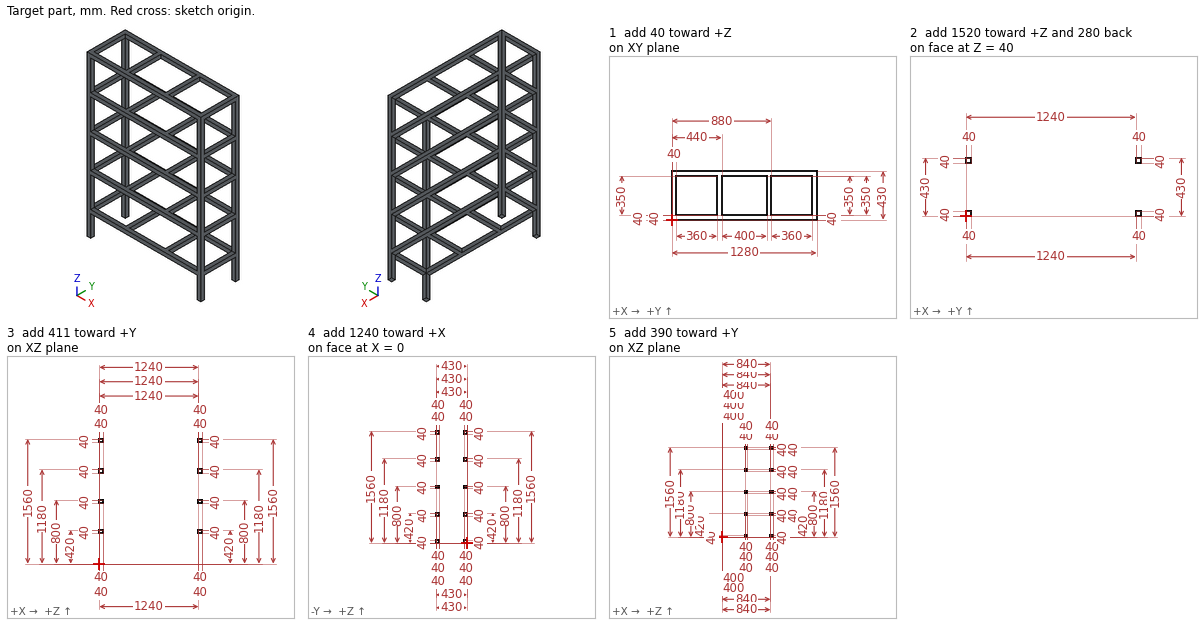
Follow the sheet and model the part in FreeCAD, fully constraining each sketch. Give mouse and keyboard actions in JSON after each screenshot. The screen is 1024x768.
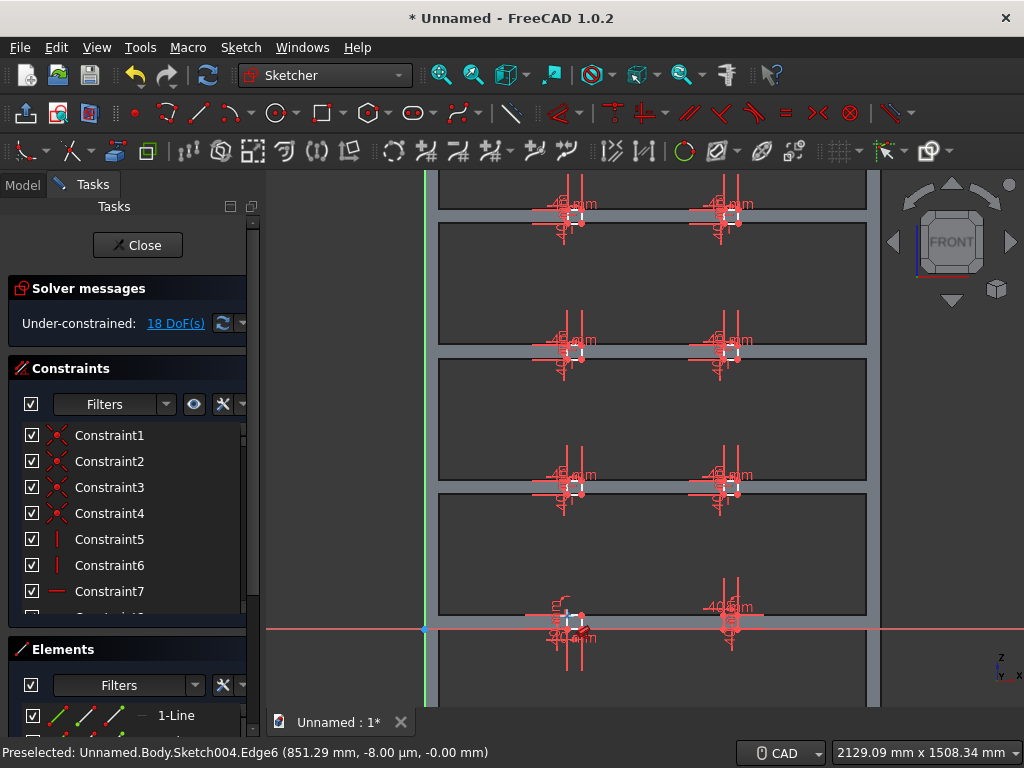
{"action": "left_click", "coordinate": [567, 615]}
{"action": "left_click", "coordinate": [496, 663]}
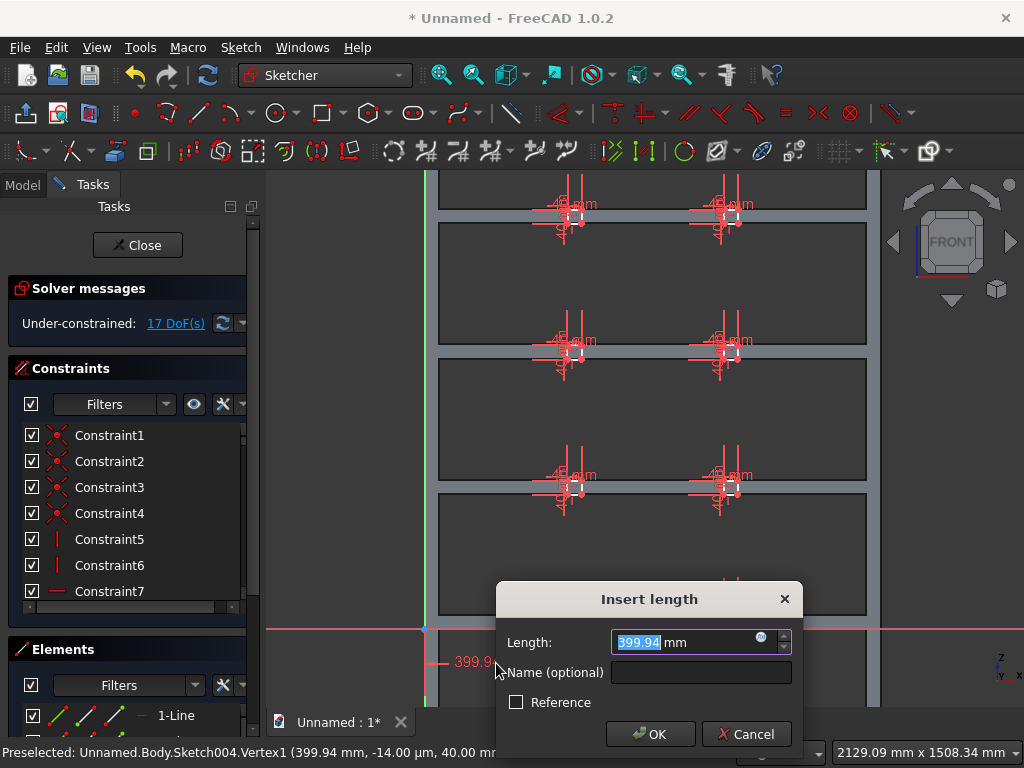
{"action": "type", "text": "400"}
{"action": "key", "text": "Return"}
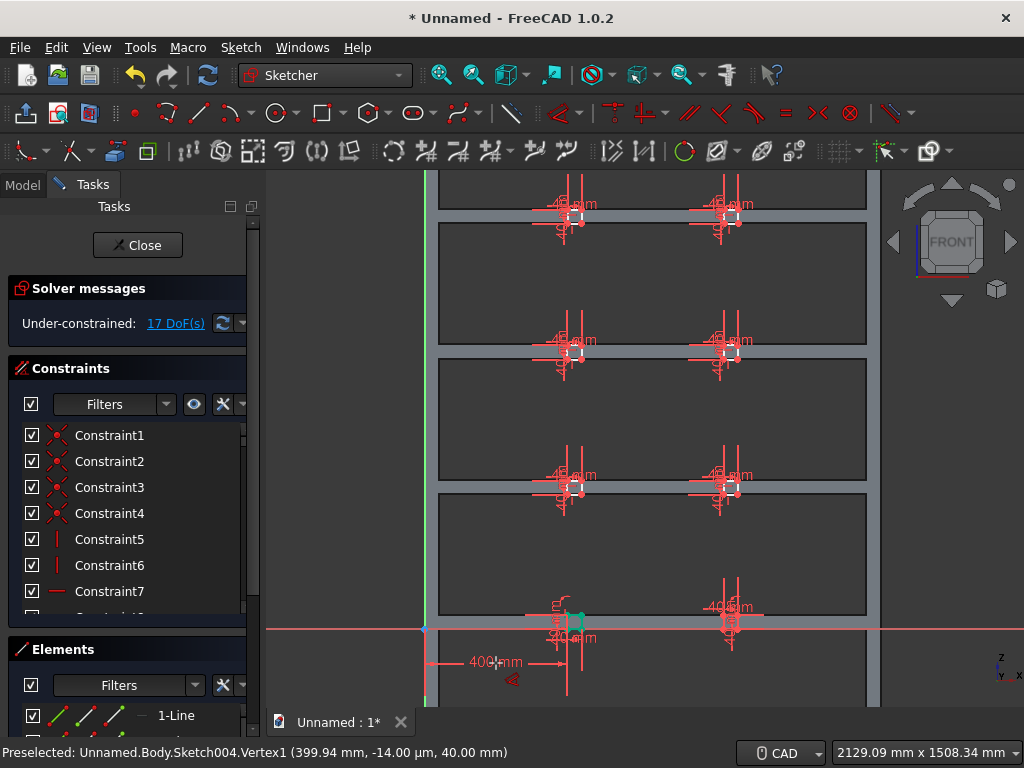
{"action": "left_click", "coordinate": [724, 615]}
{"action": "left_click", "coordinate": [574, 663]}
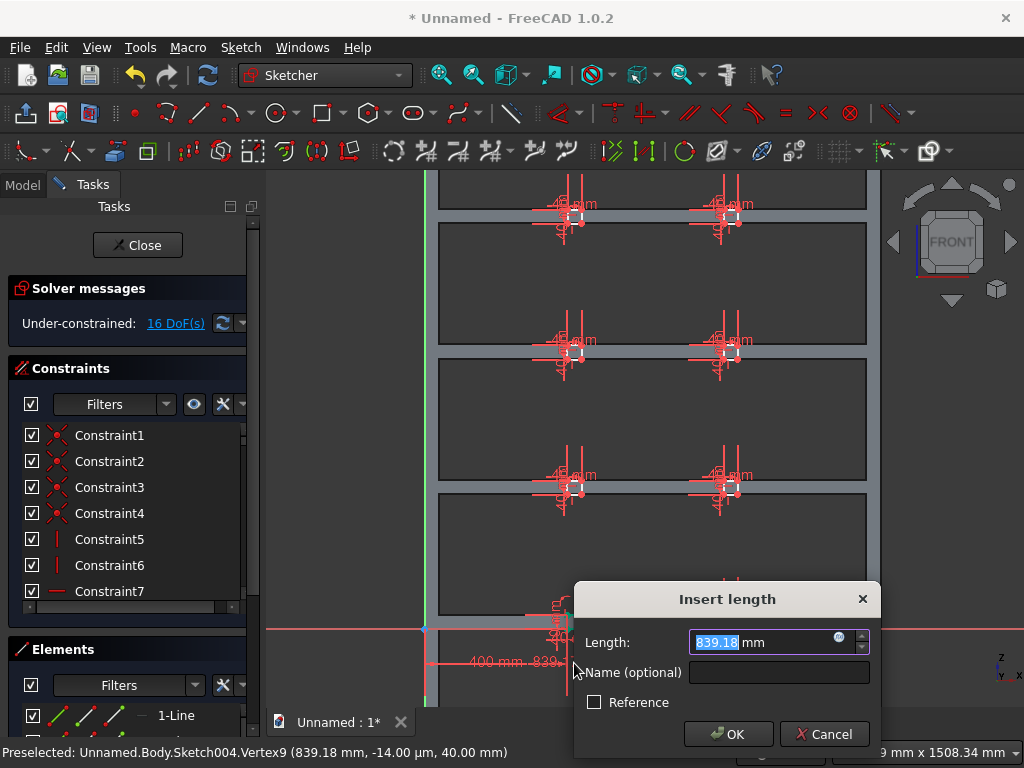
{"action": "type", "text": "840"}
{"action": "key", "text": "Return"}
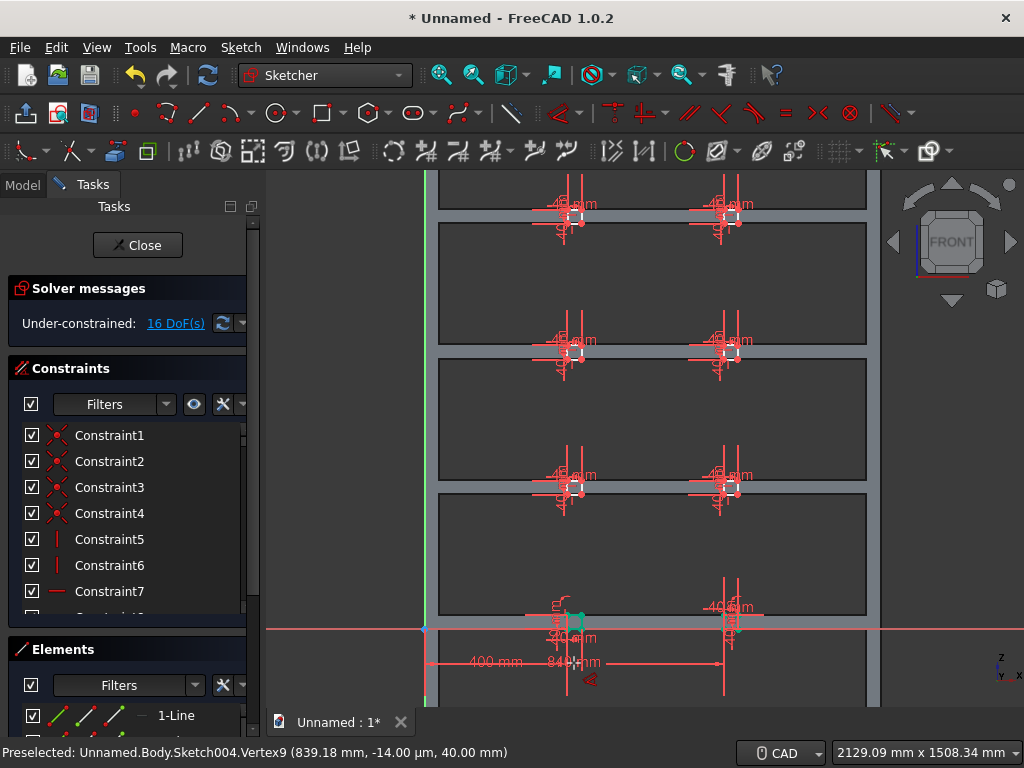
{"action": "left_click", "coordinate": [567, 481]}
{"action": "left_click", "coordinate": [496, 447]}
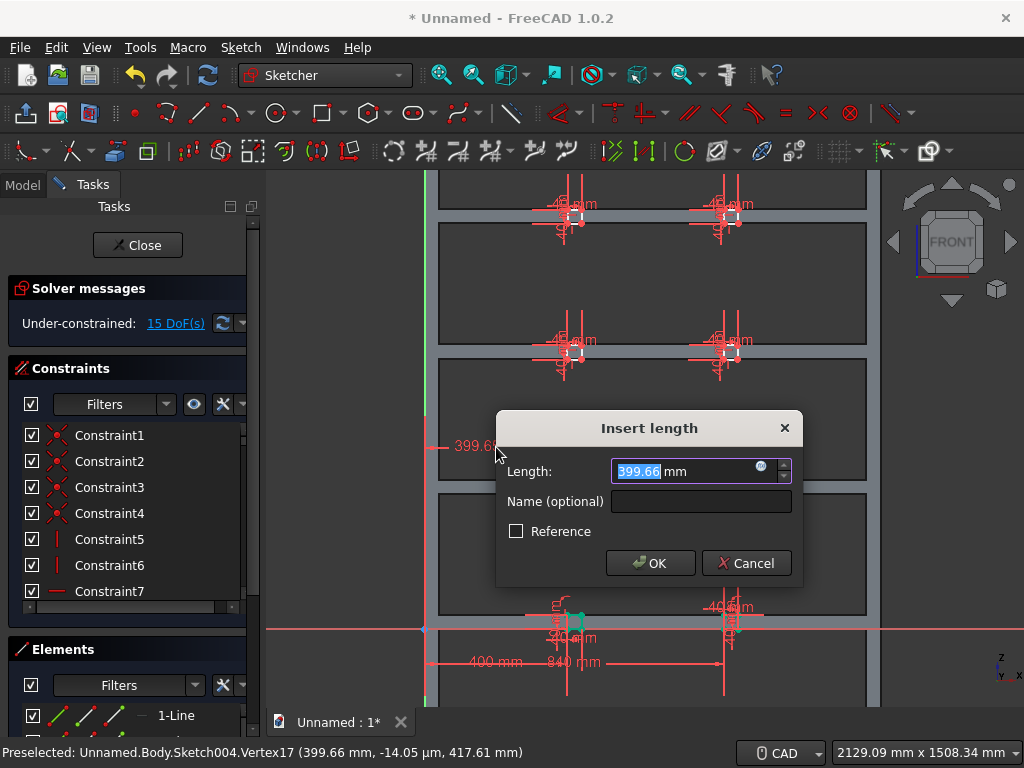
{"action": "type", "text": "400"}
{"action": "key", "text": "Return"}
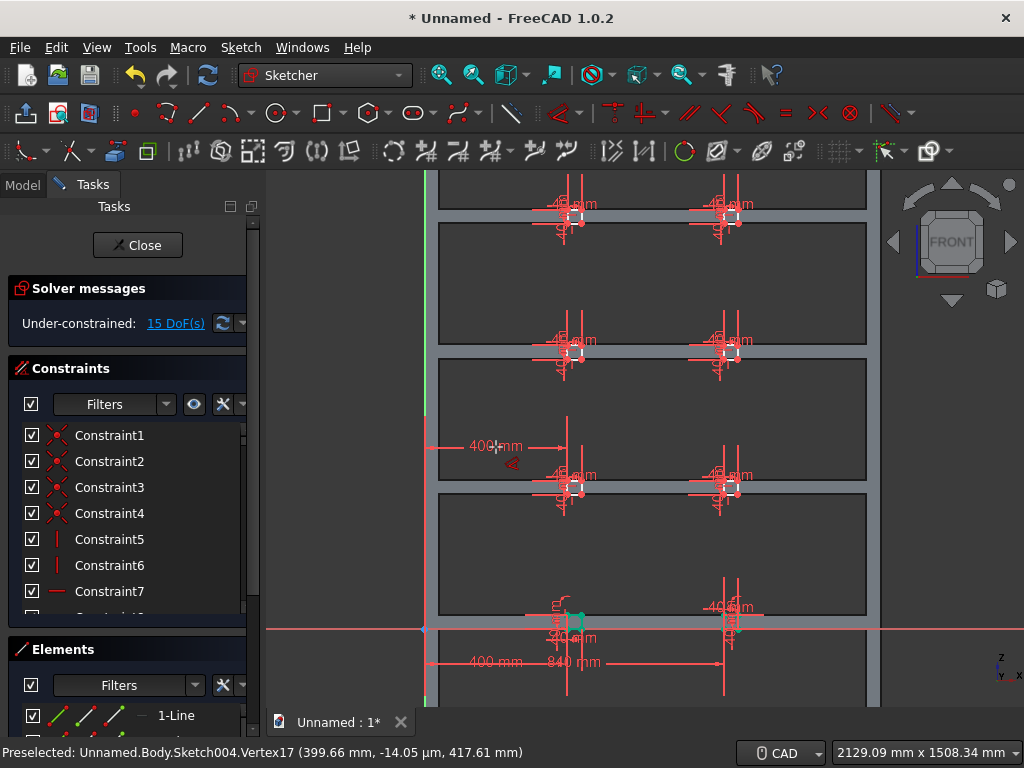
{"action": "left_click", "coordinate": [567, 481]}
{"action": "left_click", "coordinate": [391, 555]}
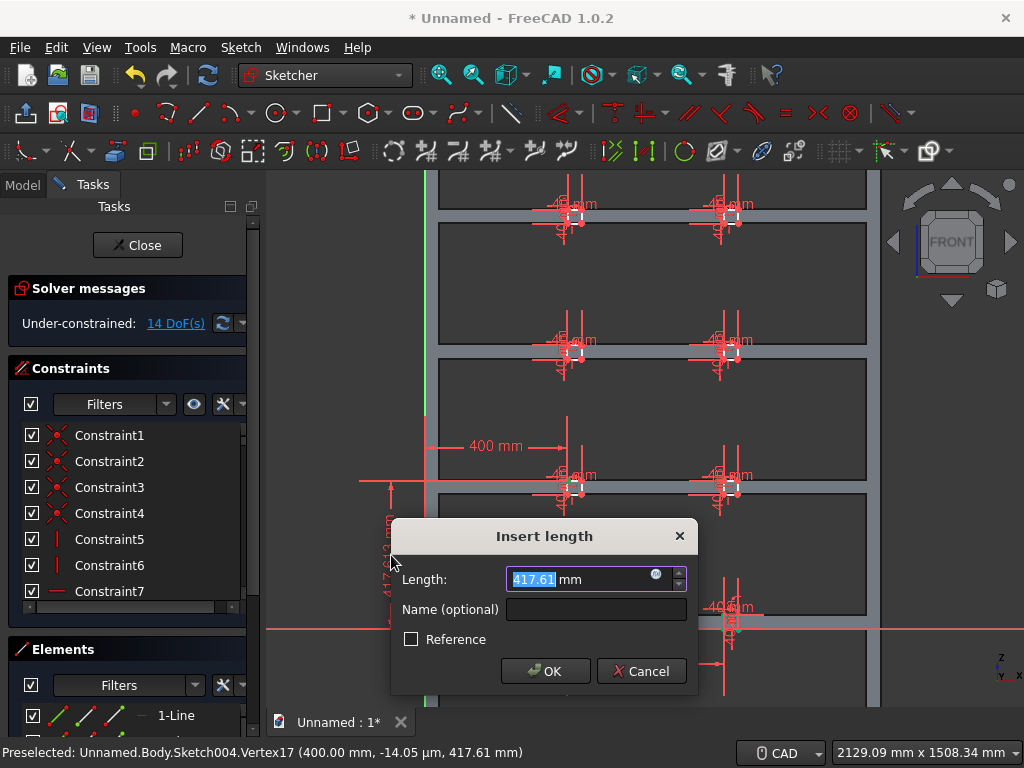
{"action": "type", "text": "420"}
{"action": "key", "text": "Return"}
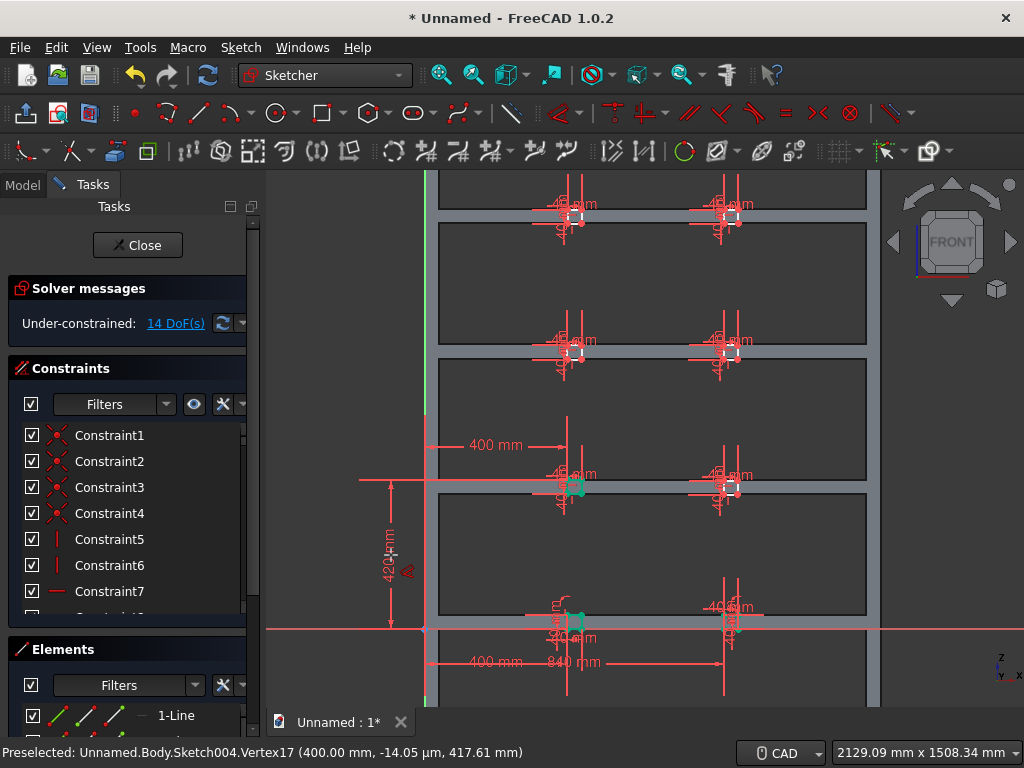
{"action": "left_click", "coordinate": [724, 481]}
{"action": "left_click", "coordinate": [679, 663]}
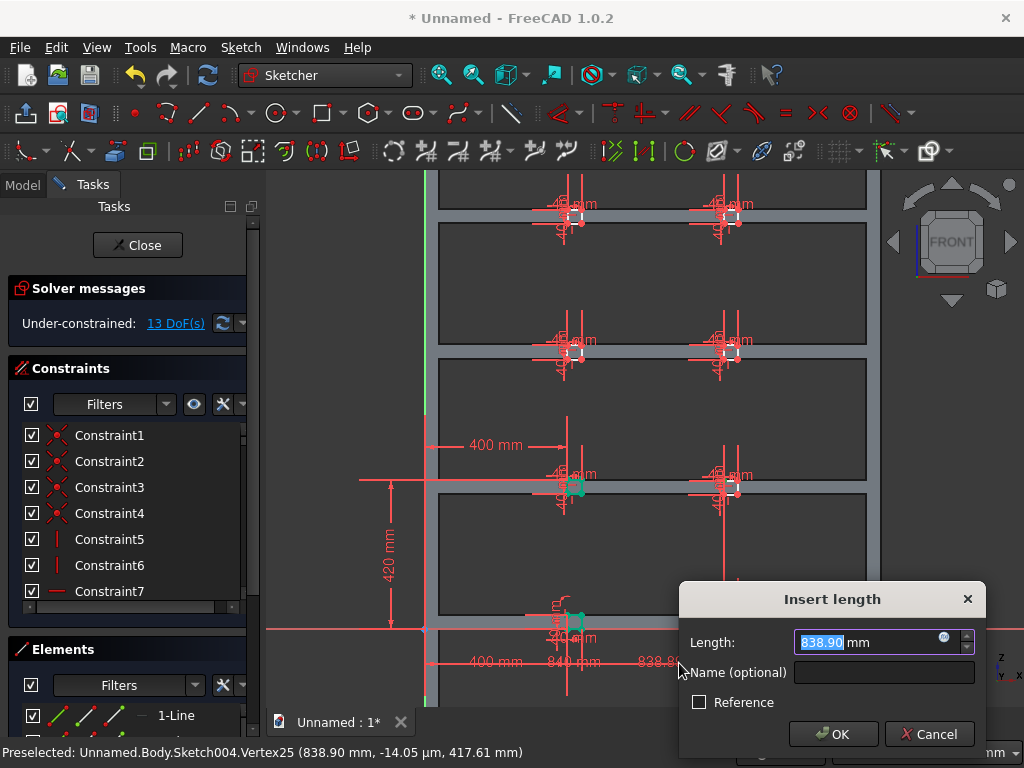
{"action": "type", "text": "840"}
{"action": "key", "text": "Return"}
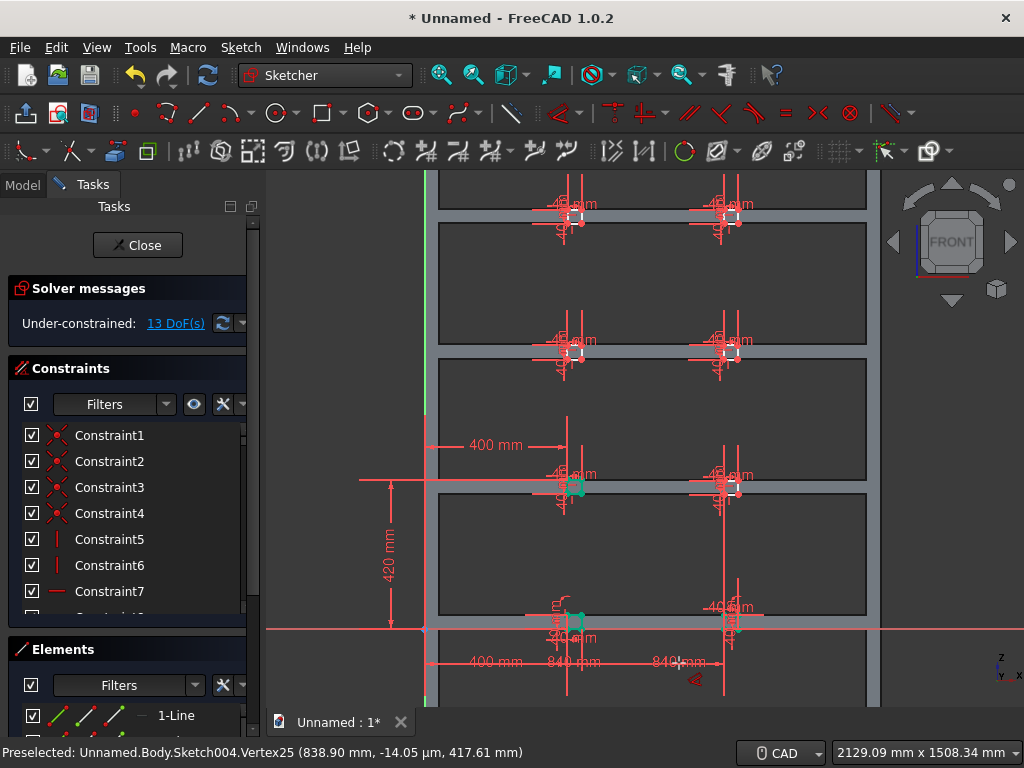
{"action": "left_click", "coordinate": [724, 481]}
{"action": "left_click", "coordinate": [391, 521]}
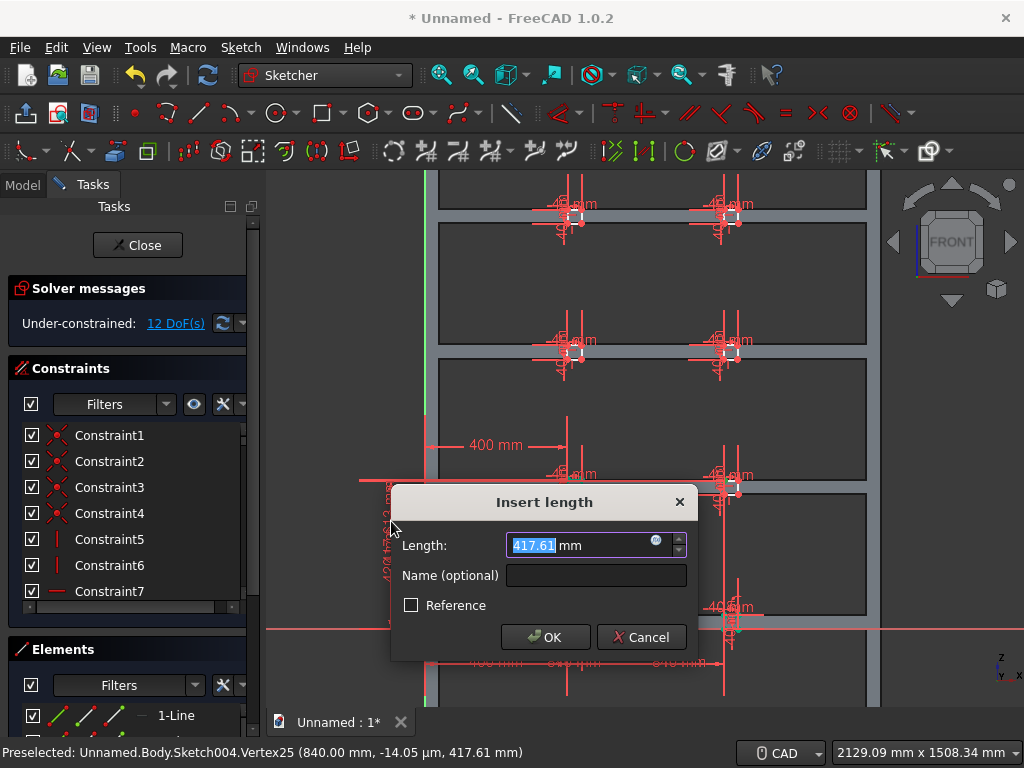
{"action": "type", "text": "420"}
{"action": "key", "text": "Return"}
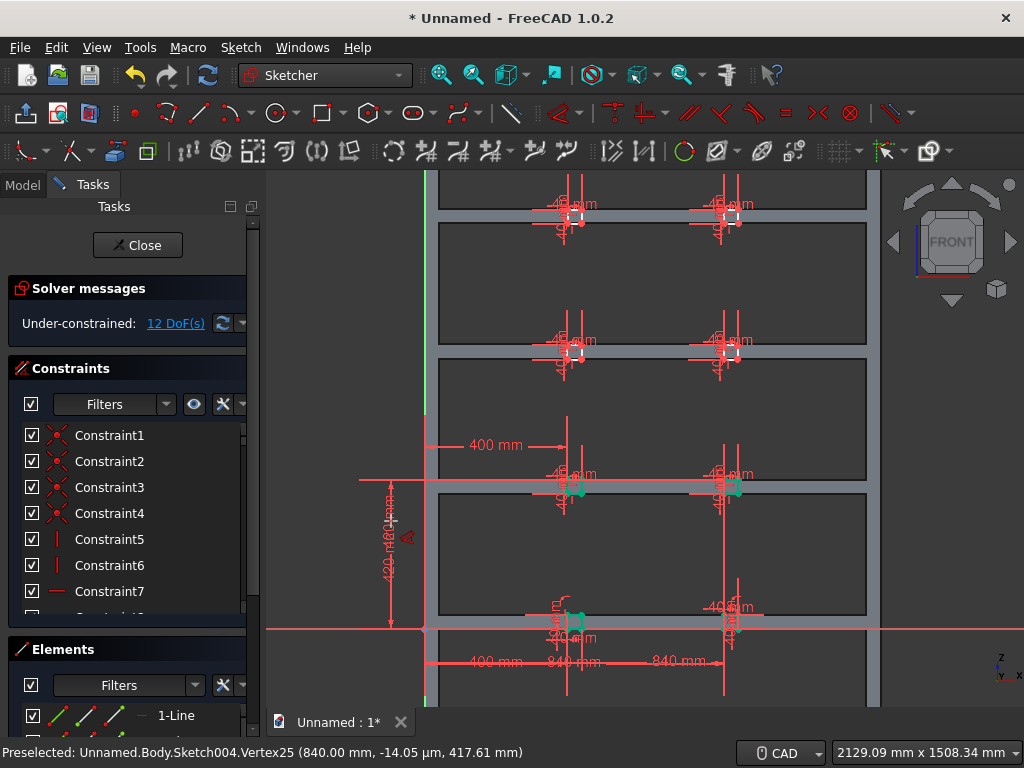
{"action": "left_click", "coordinate": [567, 345]}
{"action": "left_click", "coordinate": [496, 311]}